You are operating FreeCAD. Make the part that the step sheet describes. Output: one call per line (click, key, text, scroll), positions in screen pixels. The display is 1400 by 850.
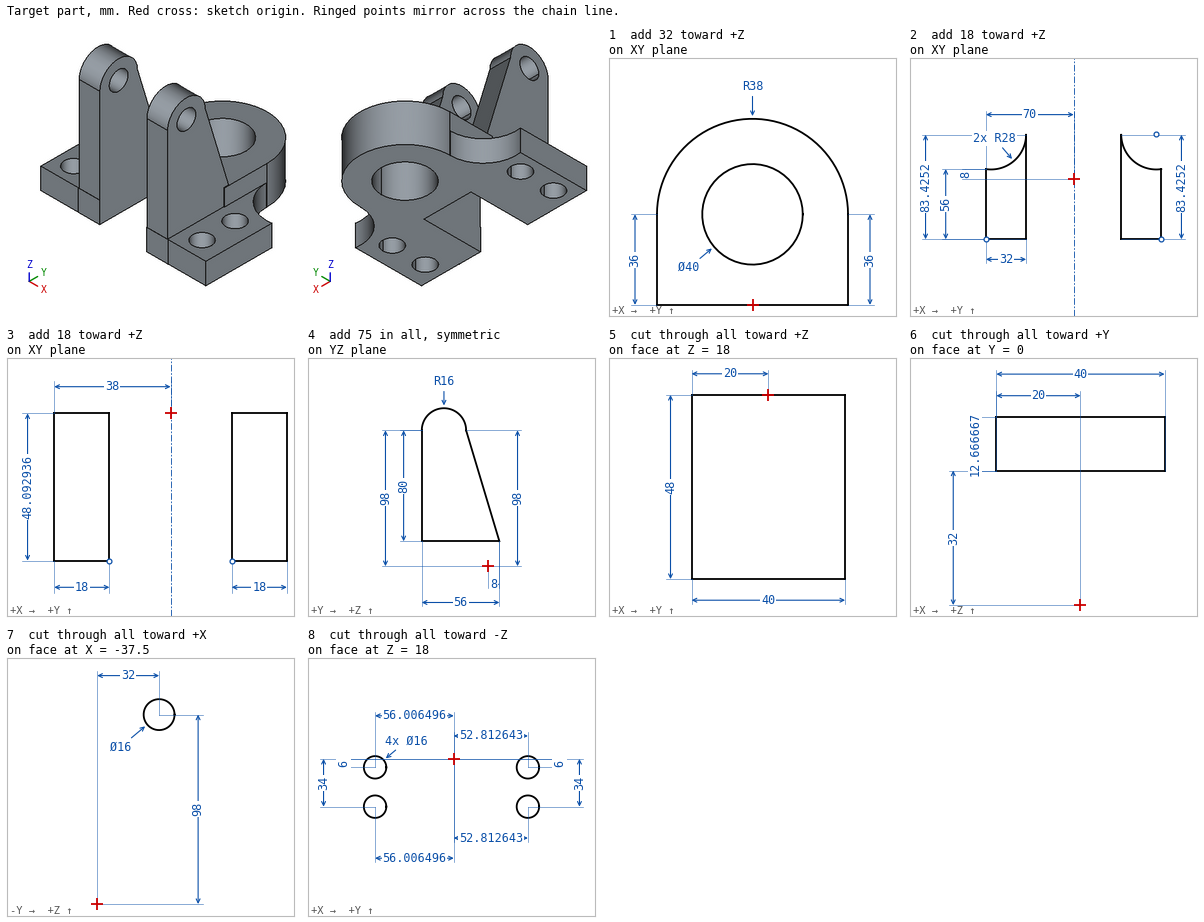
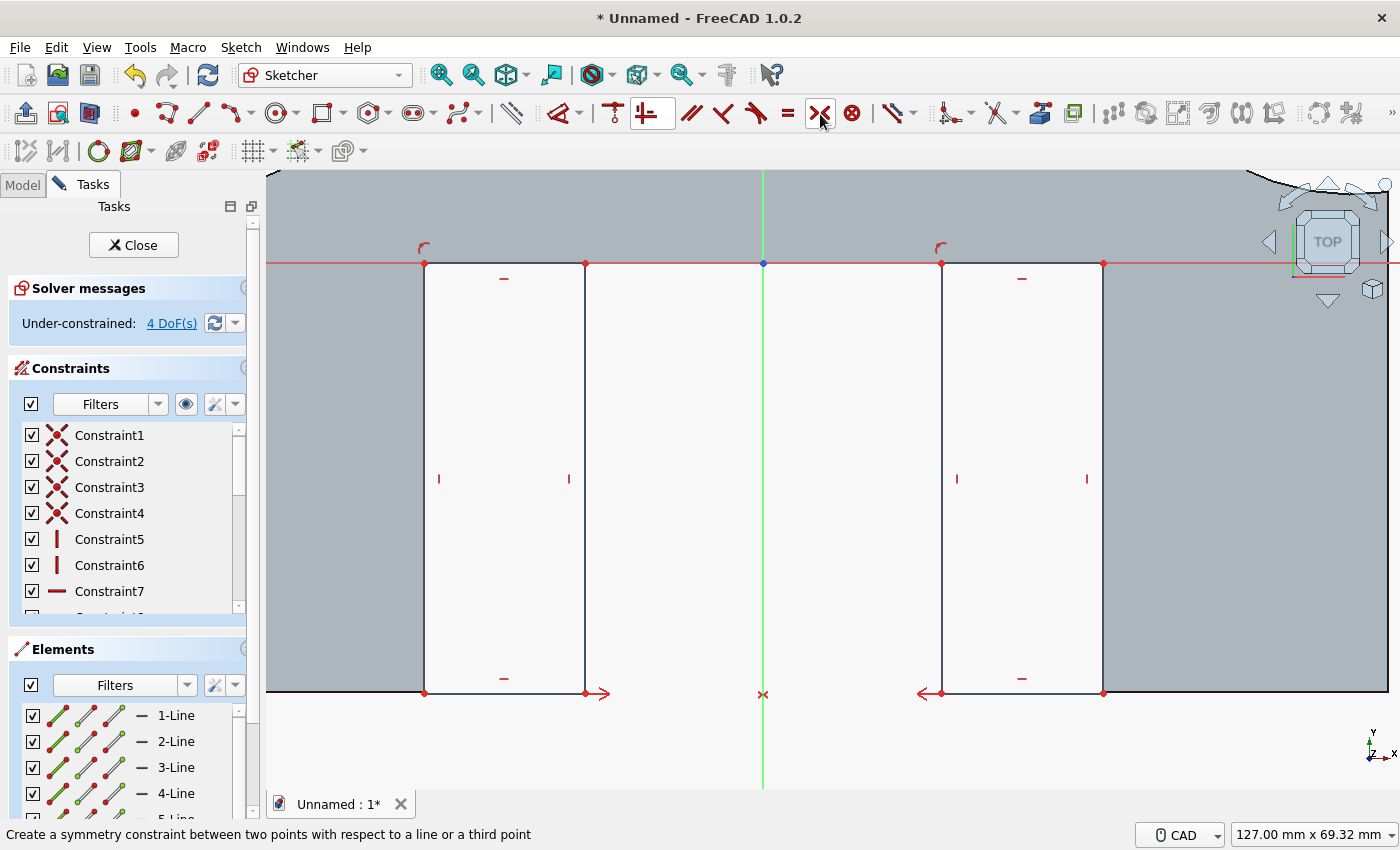
click(558, 114)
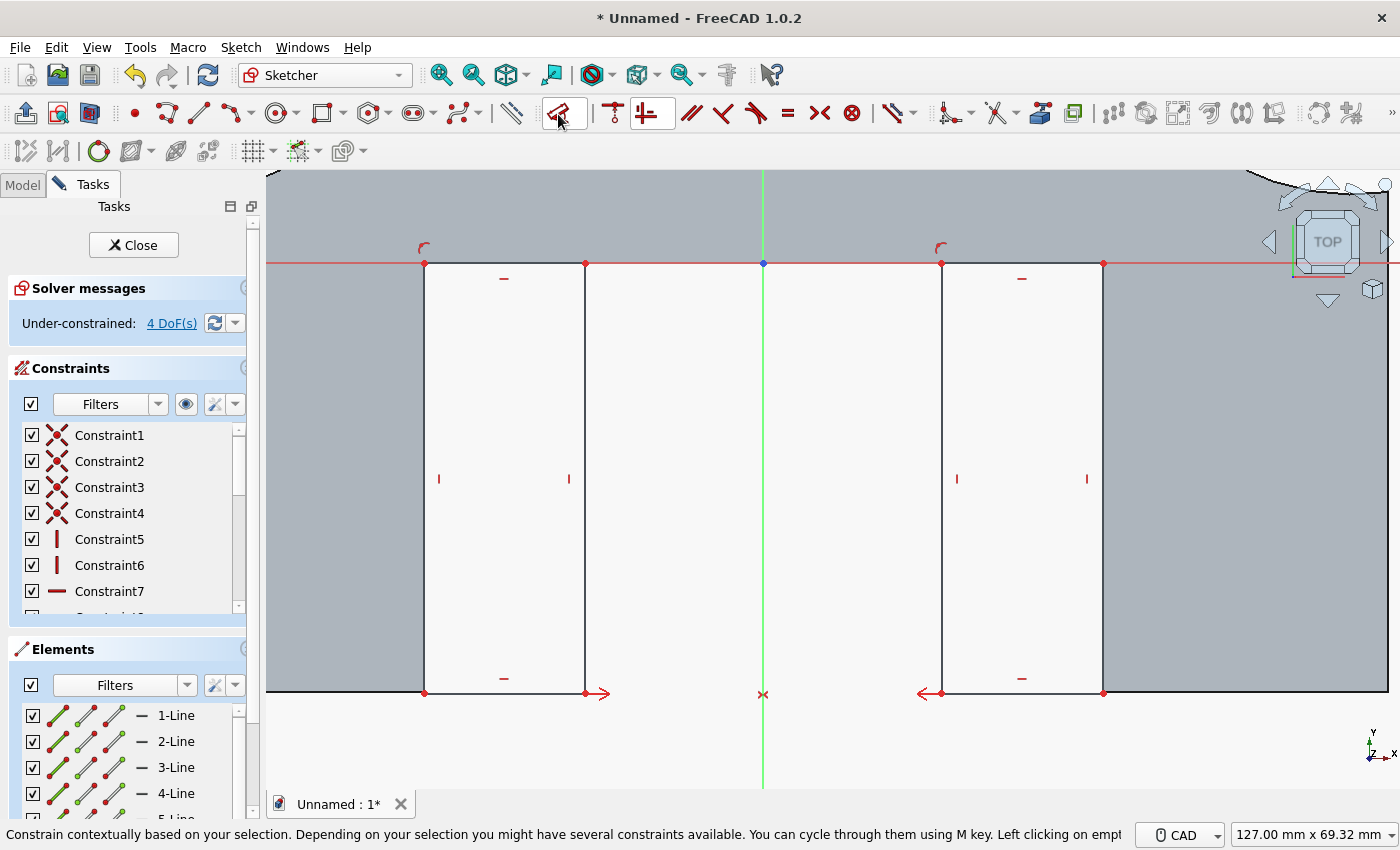
click(472, 694)
click(505, 728)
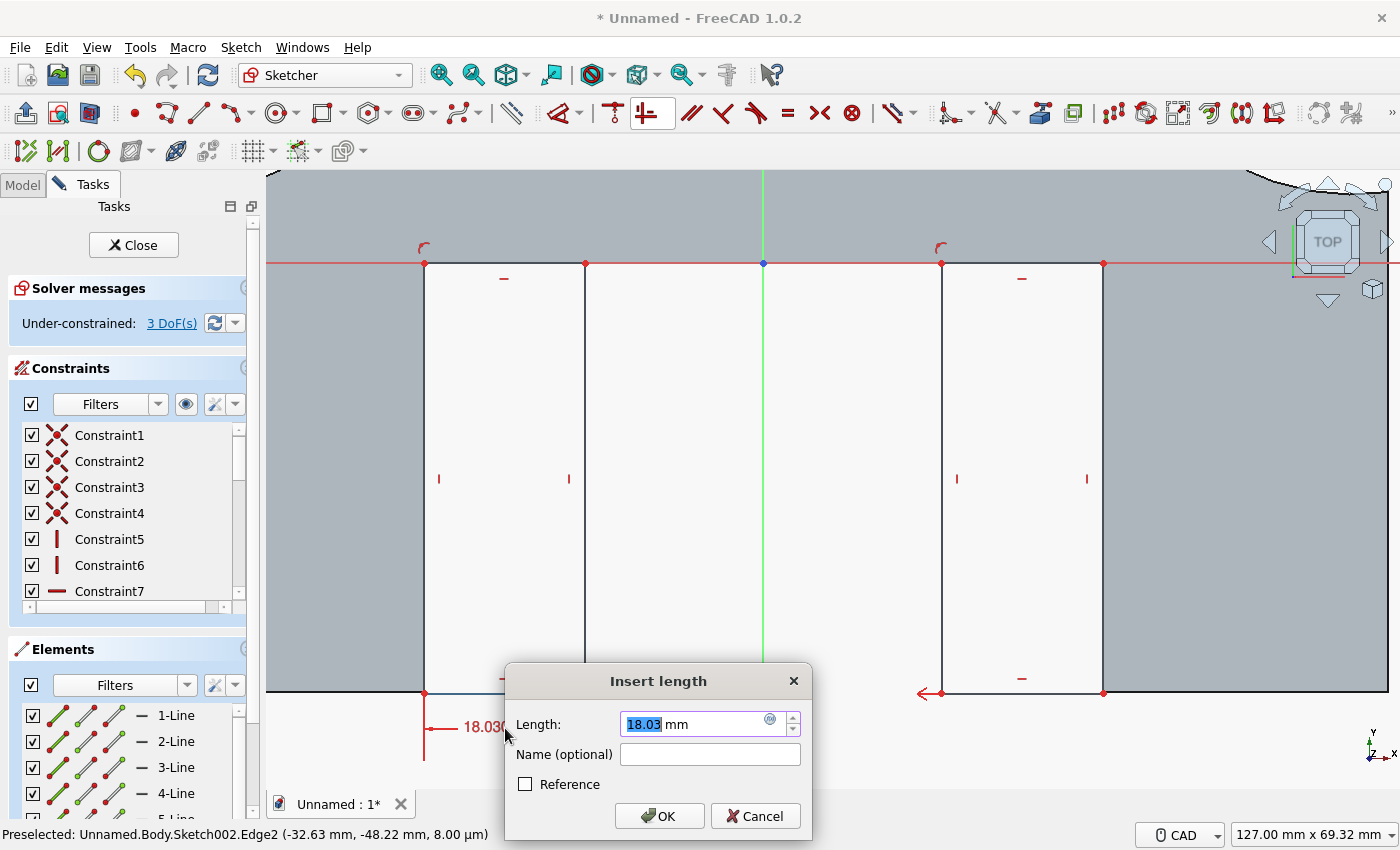
text(18)
key(Return)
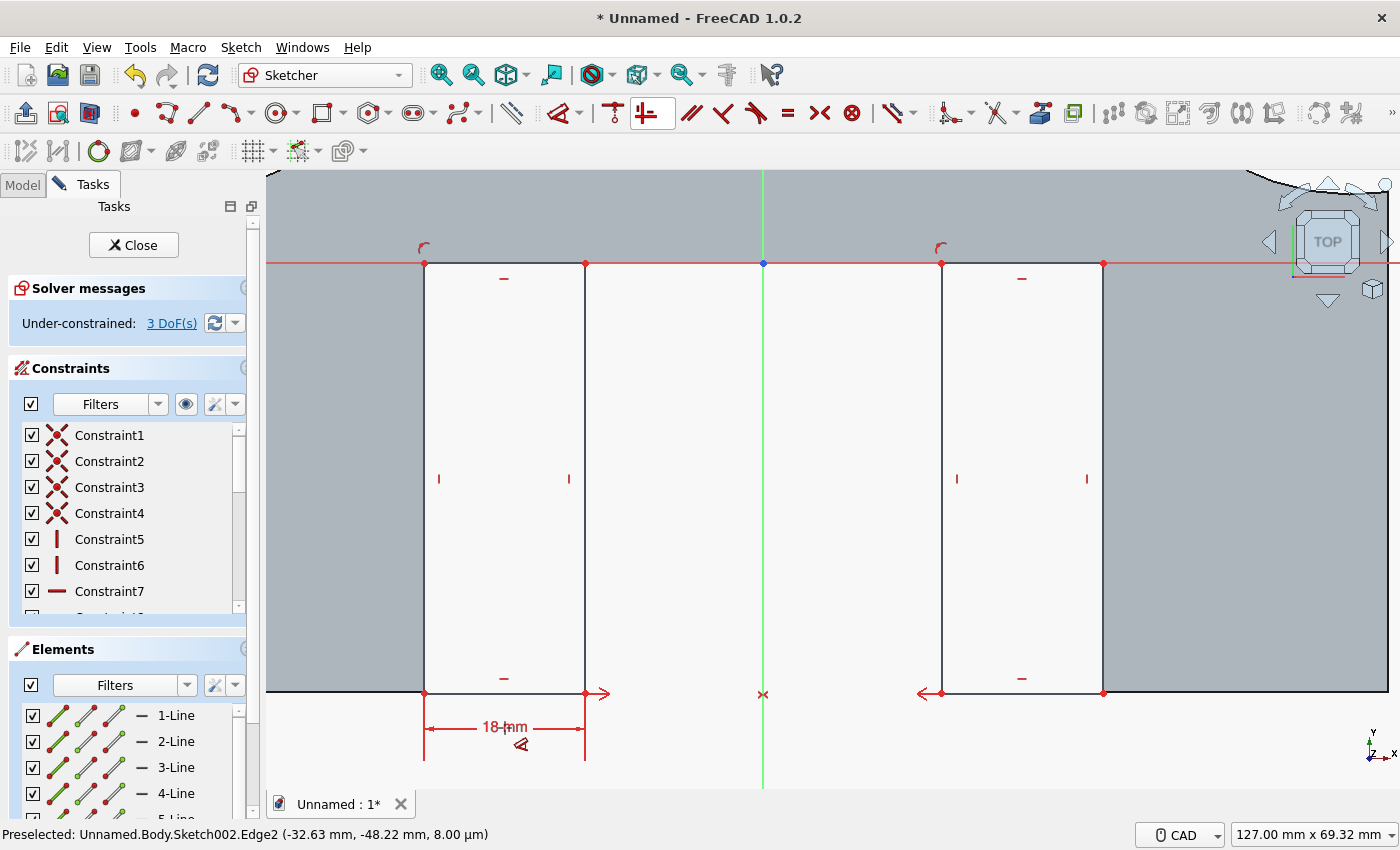
click(990, 694)
click(1022, 728)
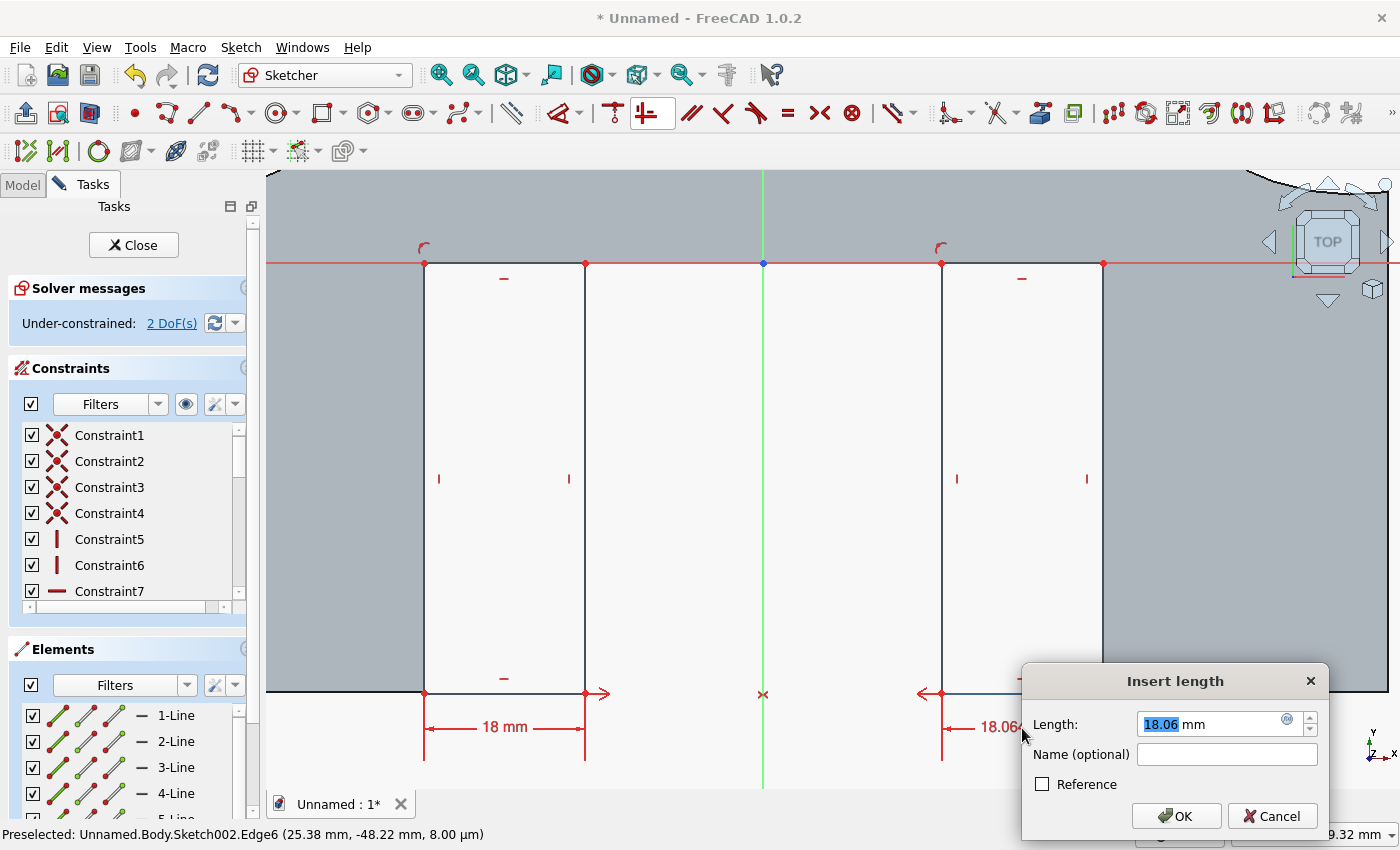
text(18)
key(Return)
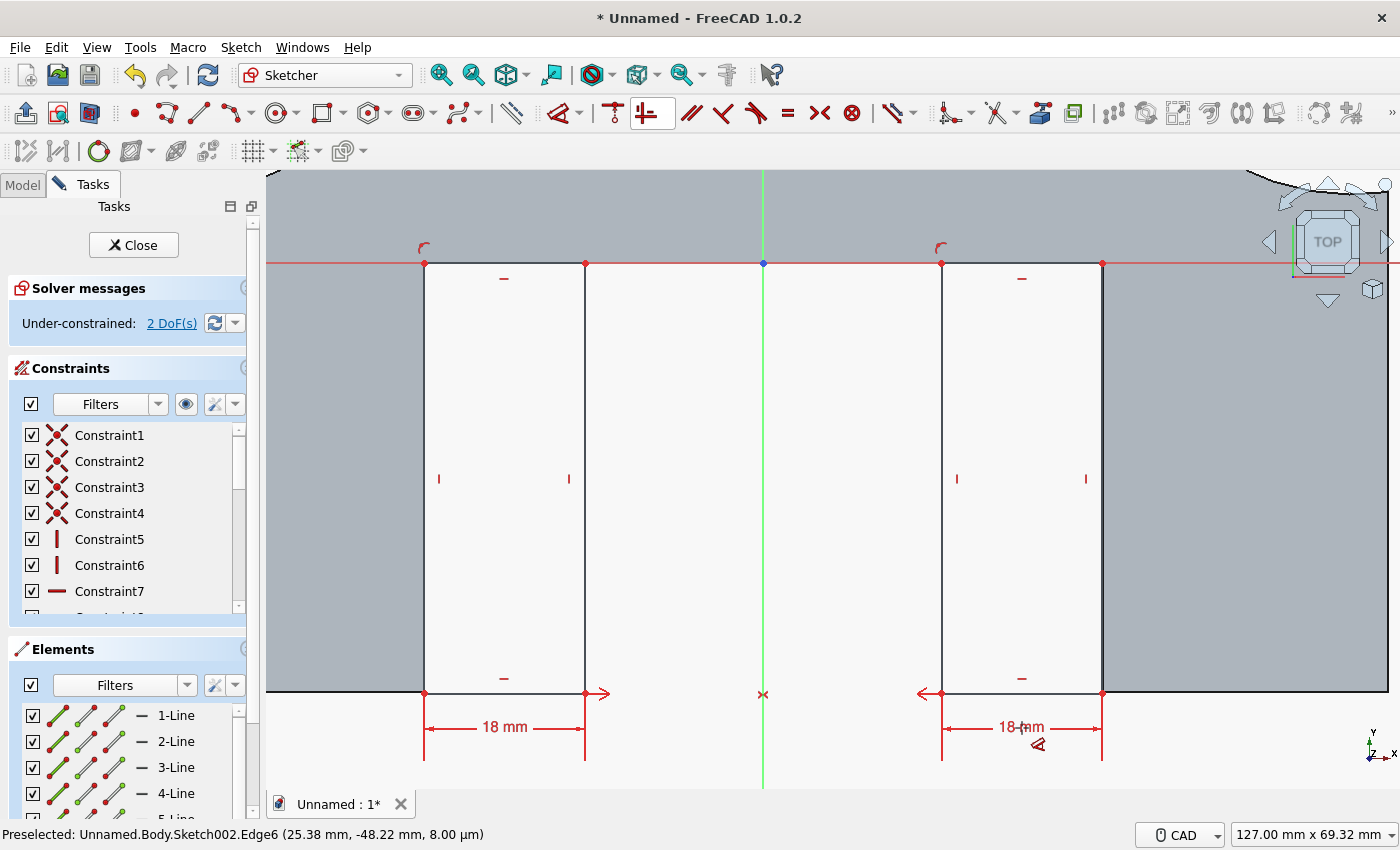
click(424, 263)
click(594, 229)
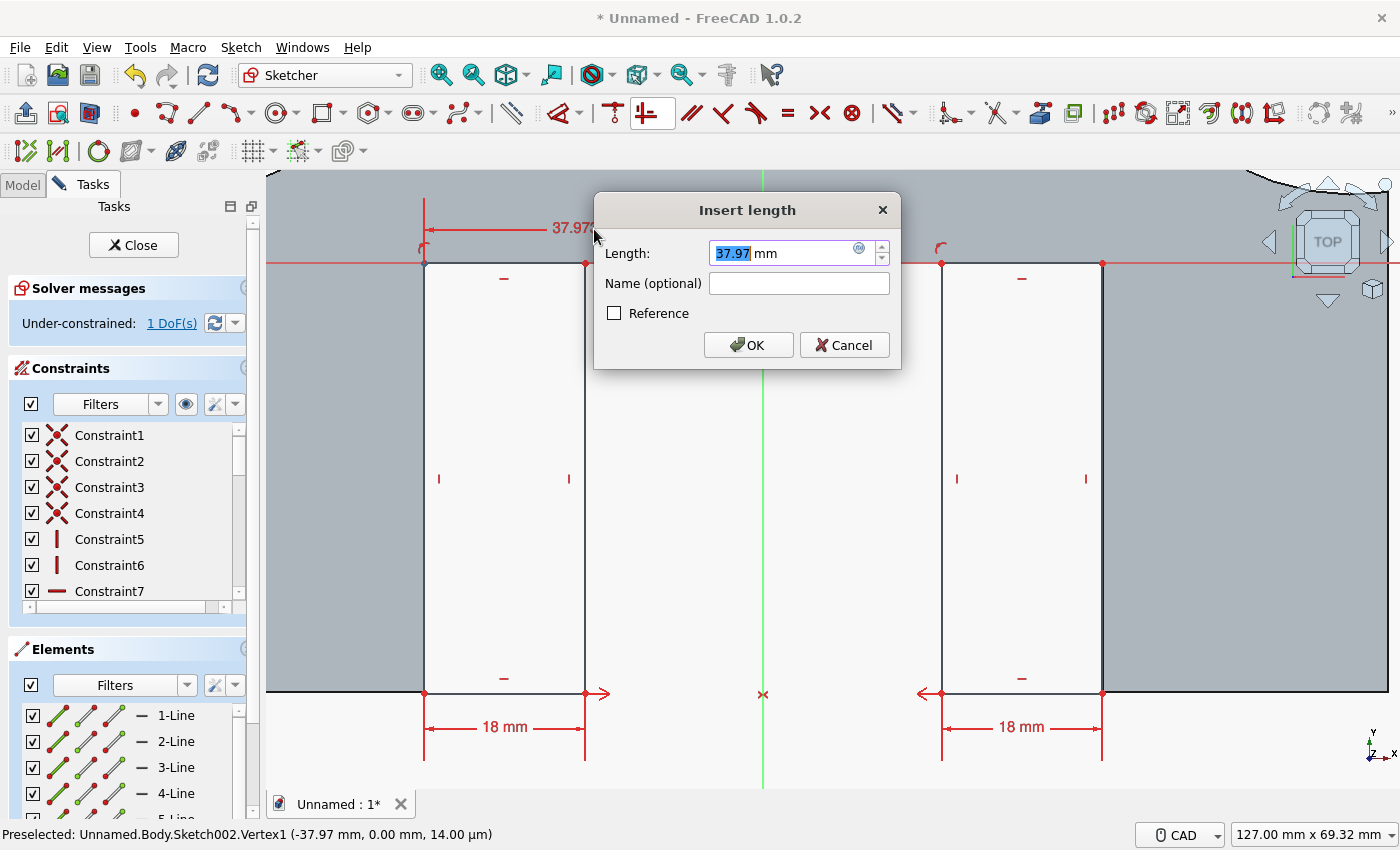
text(38)
key(Return)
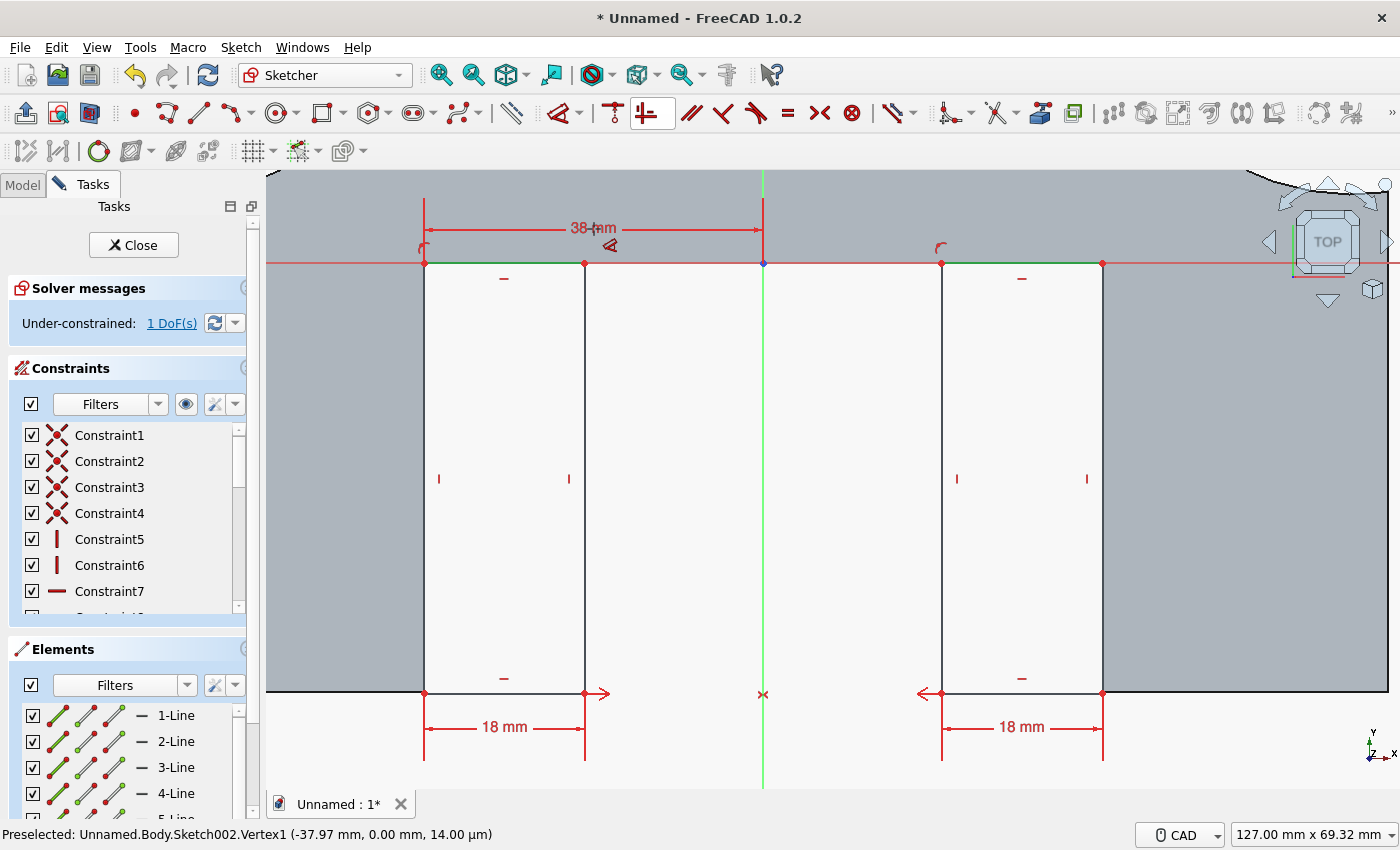
click(424, 393)
click(390, 479)